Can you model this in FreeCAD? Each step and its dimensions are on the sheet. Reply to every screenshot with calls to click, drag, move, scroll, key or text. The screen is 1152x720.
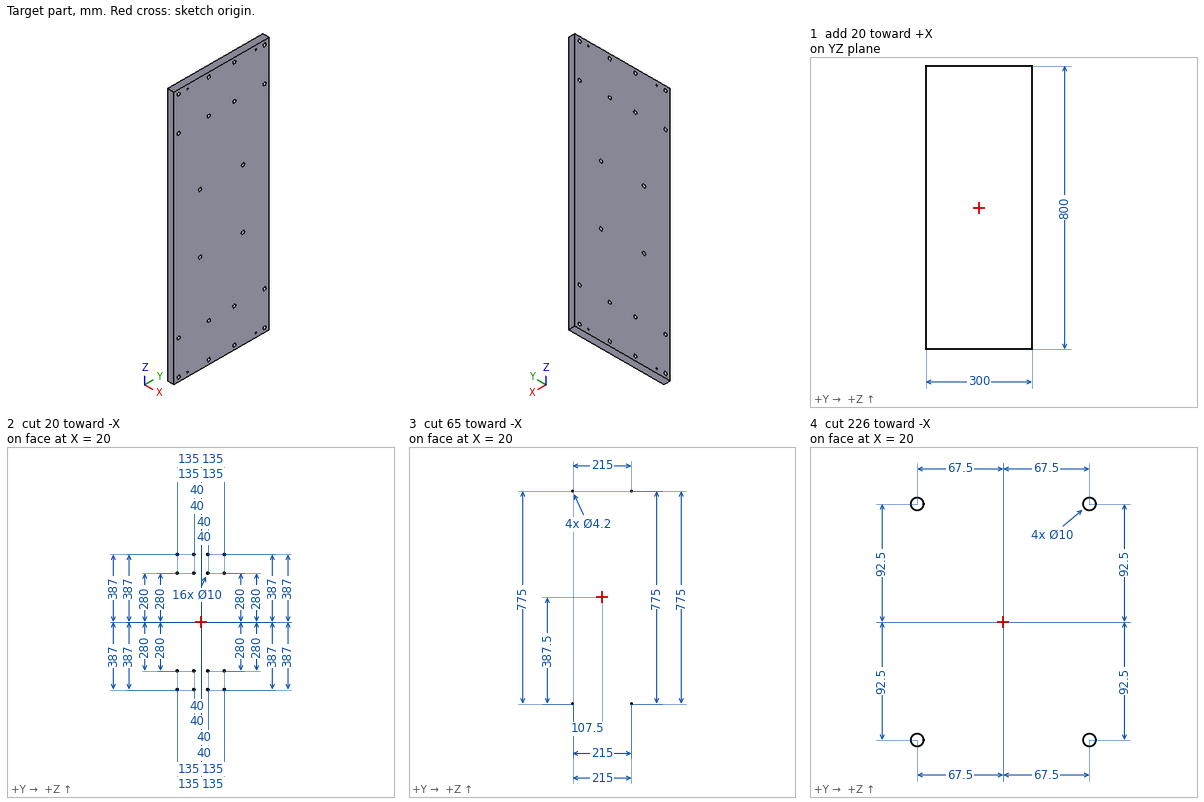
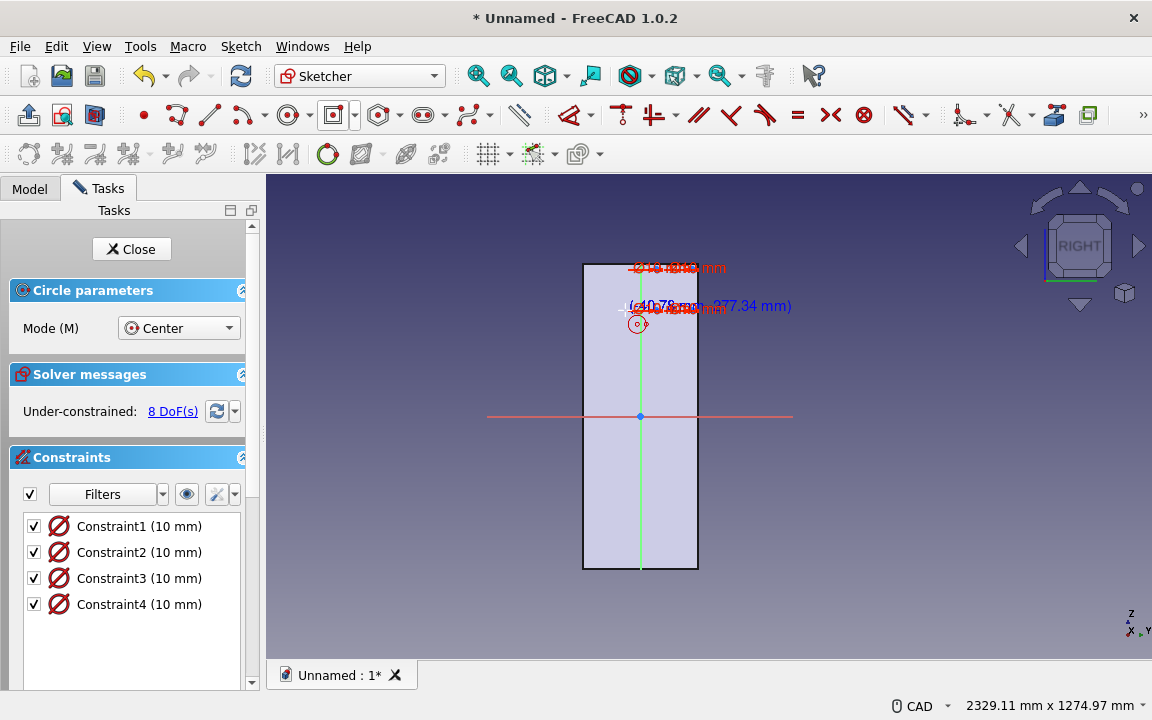
click(625, 310)
move(624, 309)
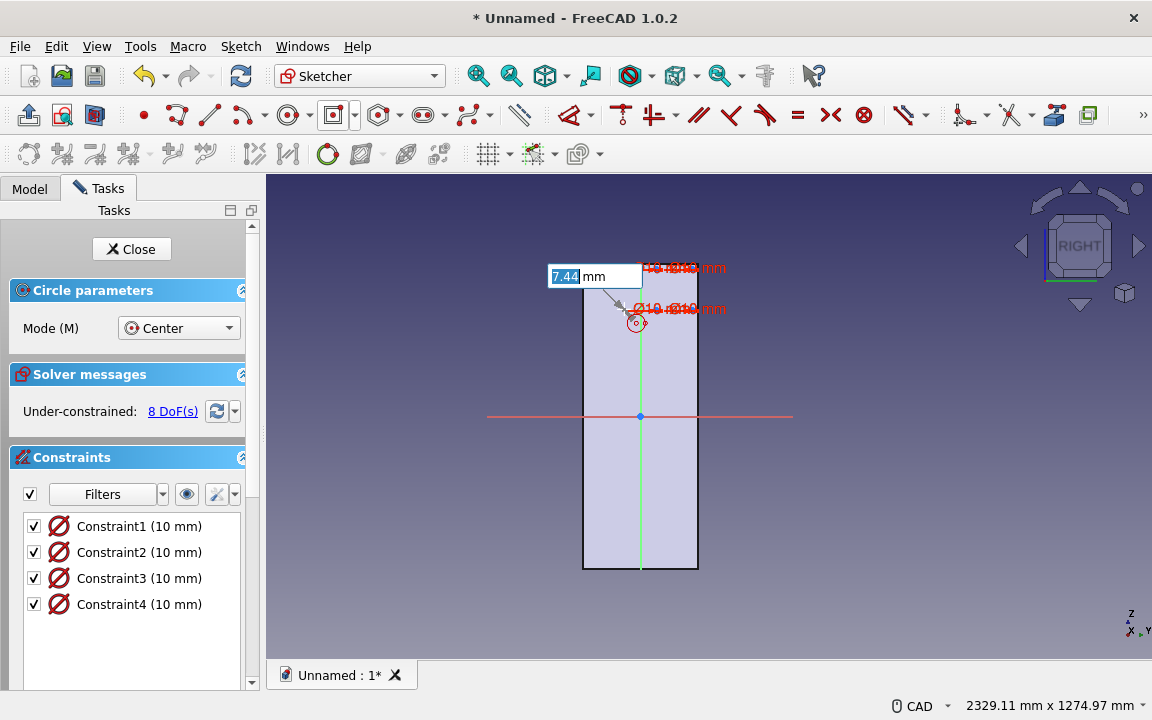
text(10)
key(Return)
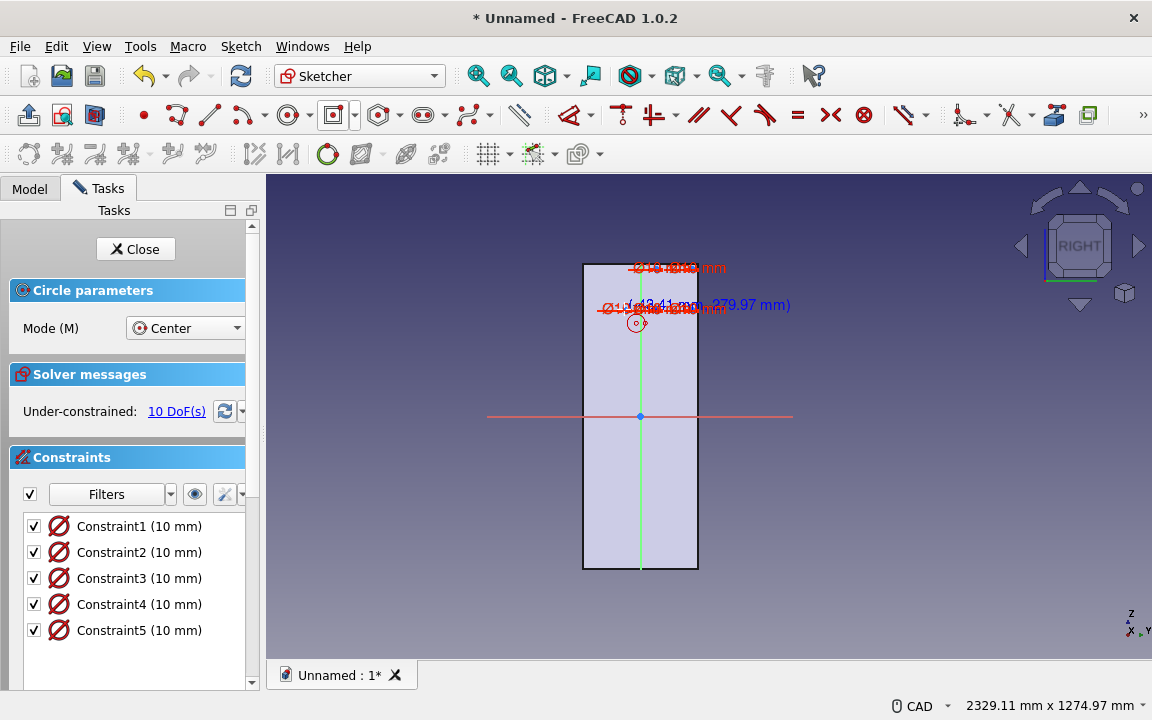
scroll(589, 310, up, 13)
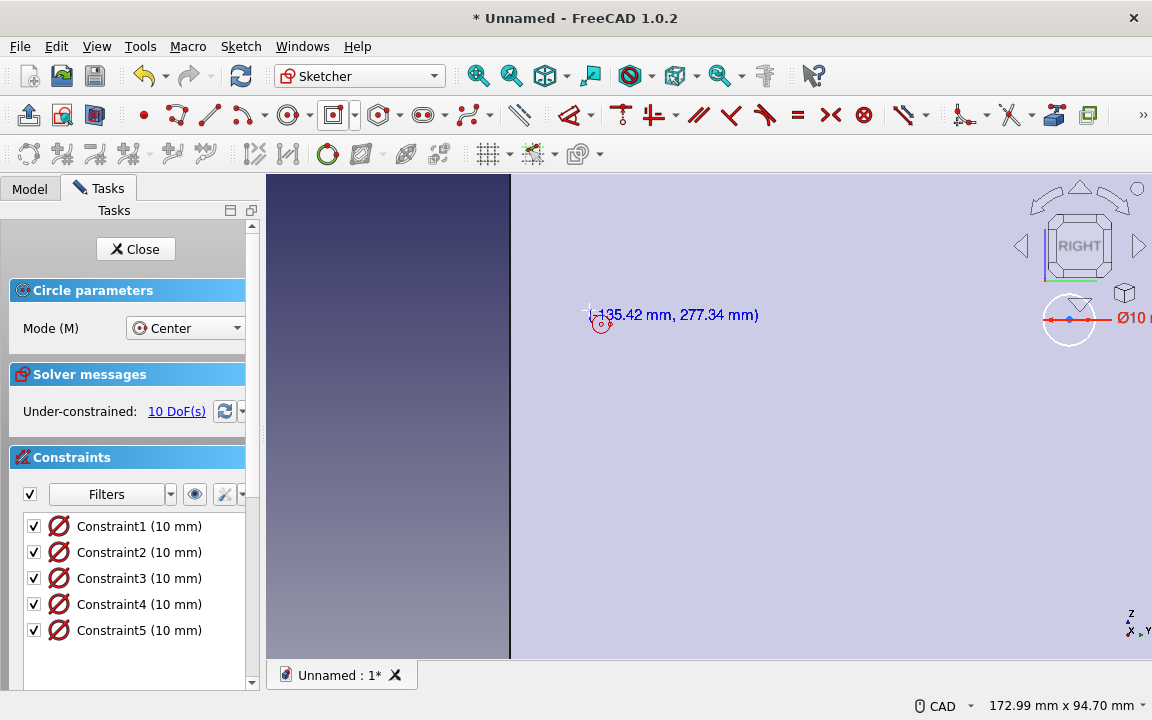
scroll(589, 310, down, 13)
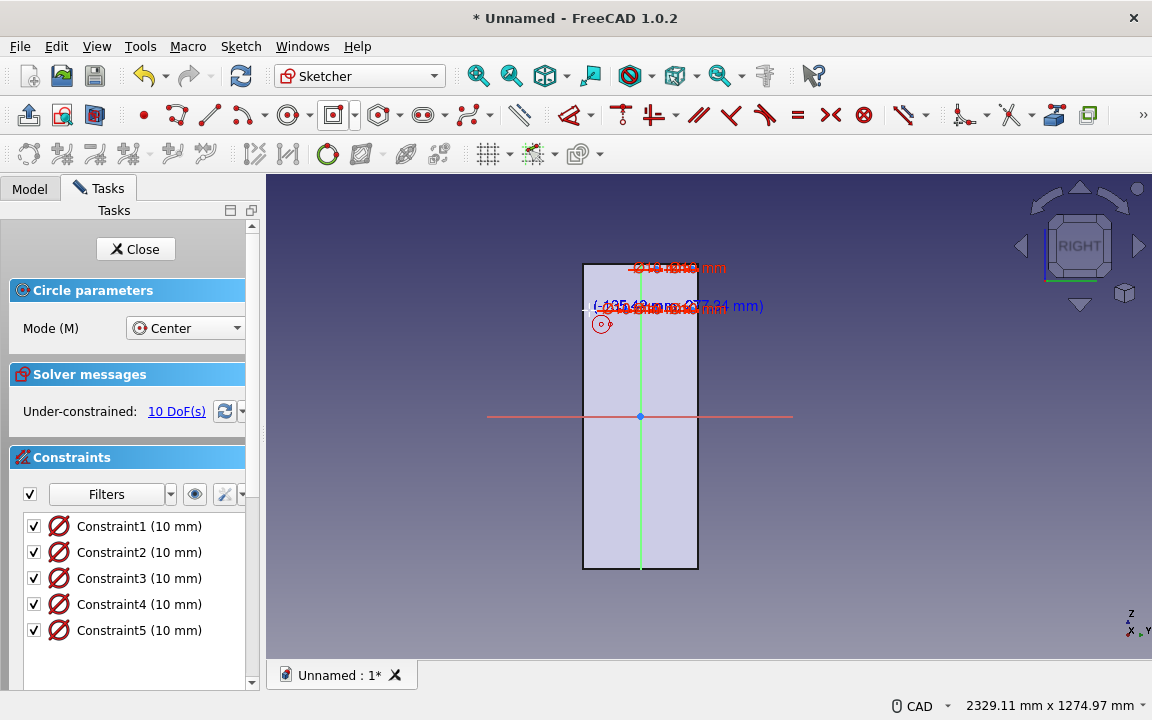
click(589, 310)
move(591, 309)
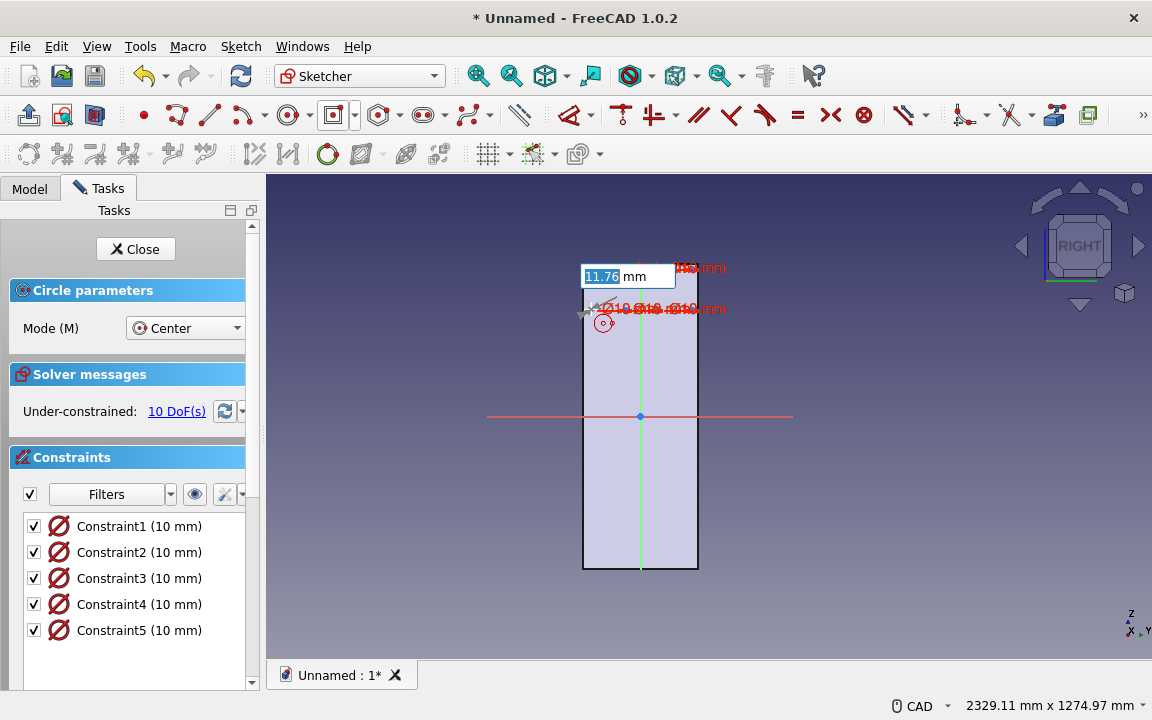
text(10)
key(Return)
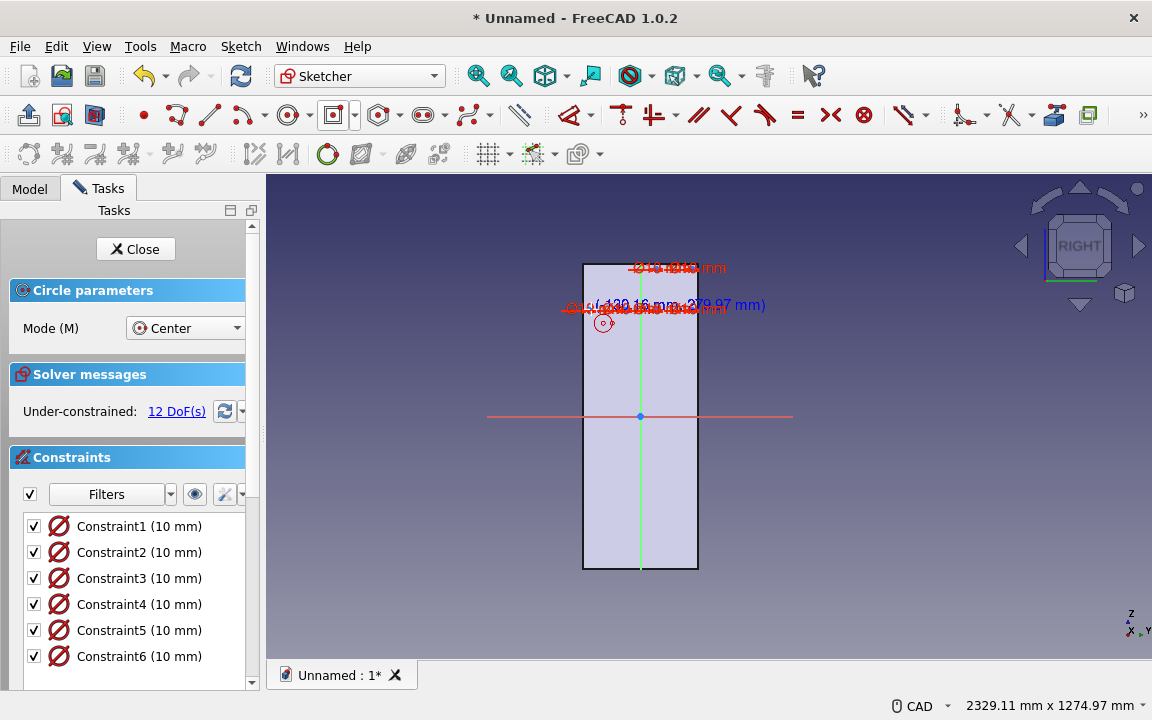
scroll(589, 269, up, 13)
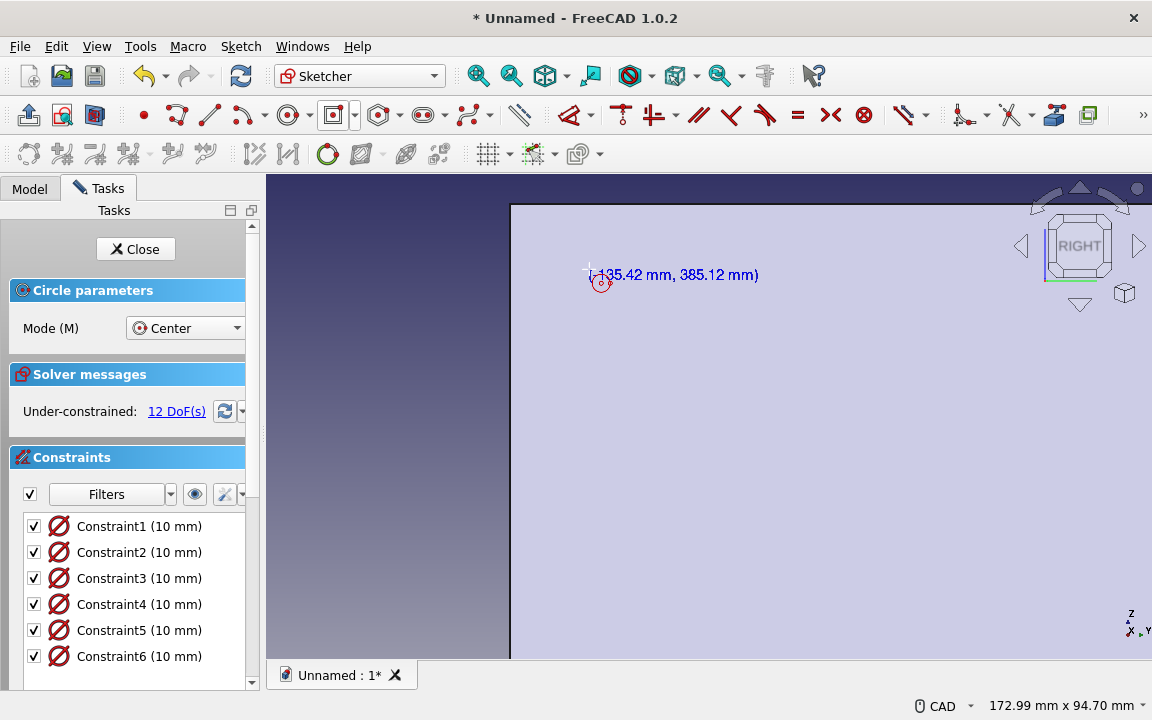
scroll(589, 269, down, 13)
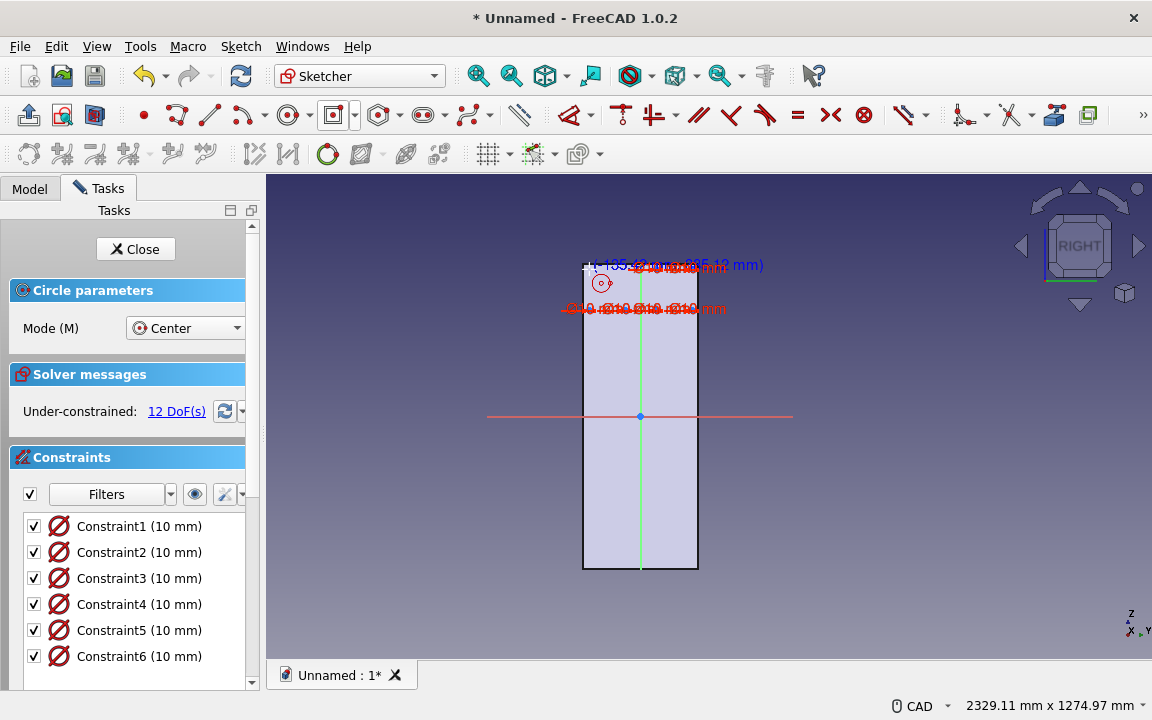
click(589, 269)
move(591, 268)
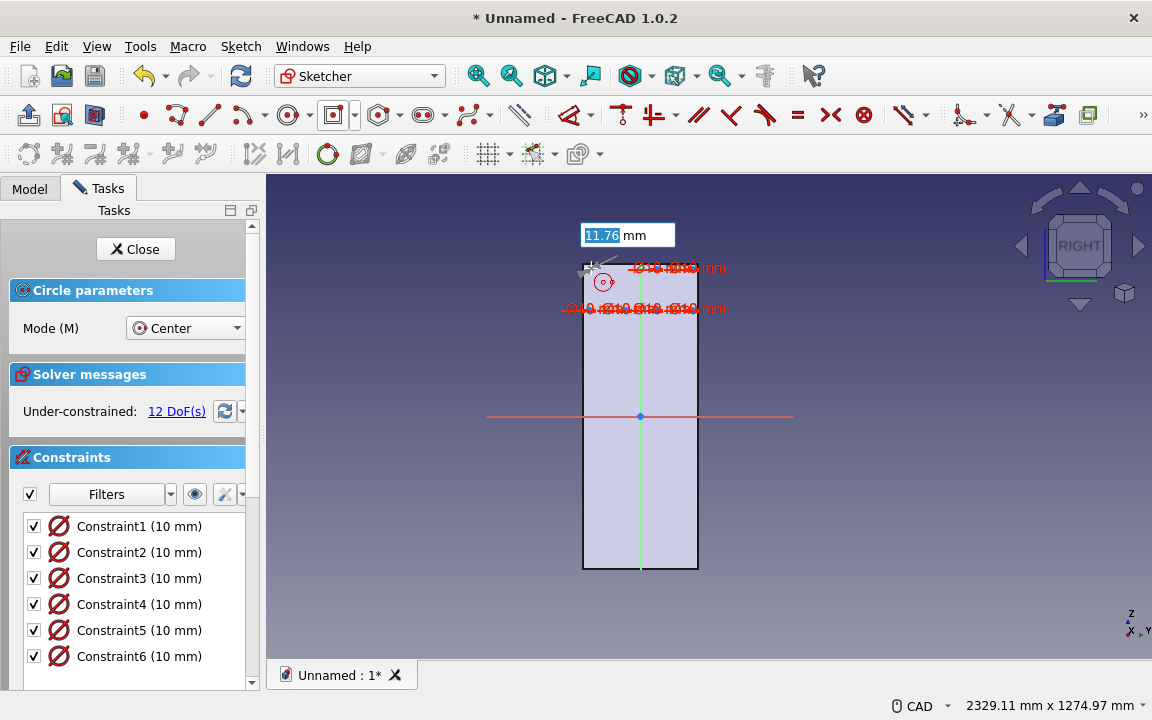
text(10)
key(Return)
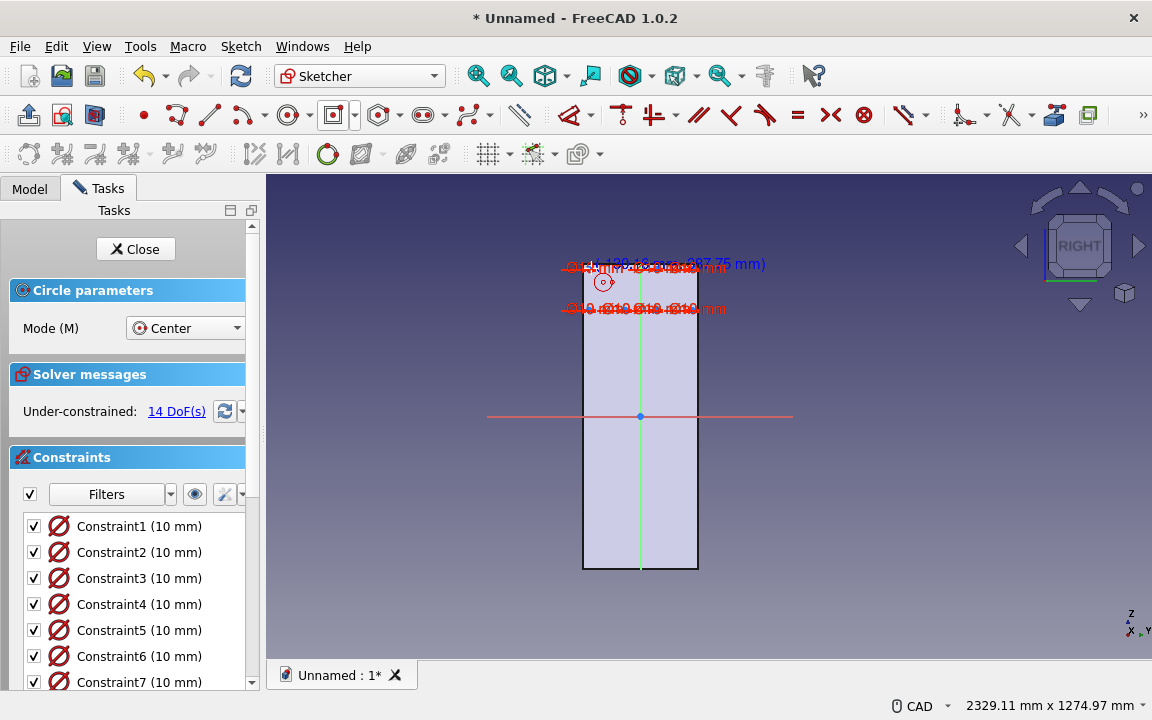
scroll(625, 269, up, 13)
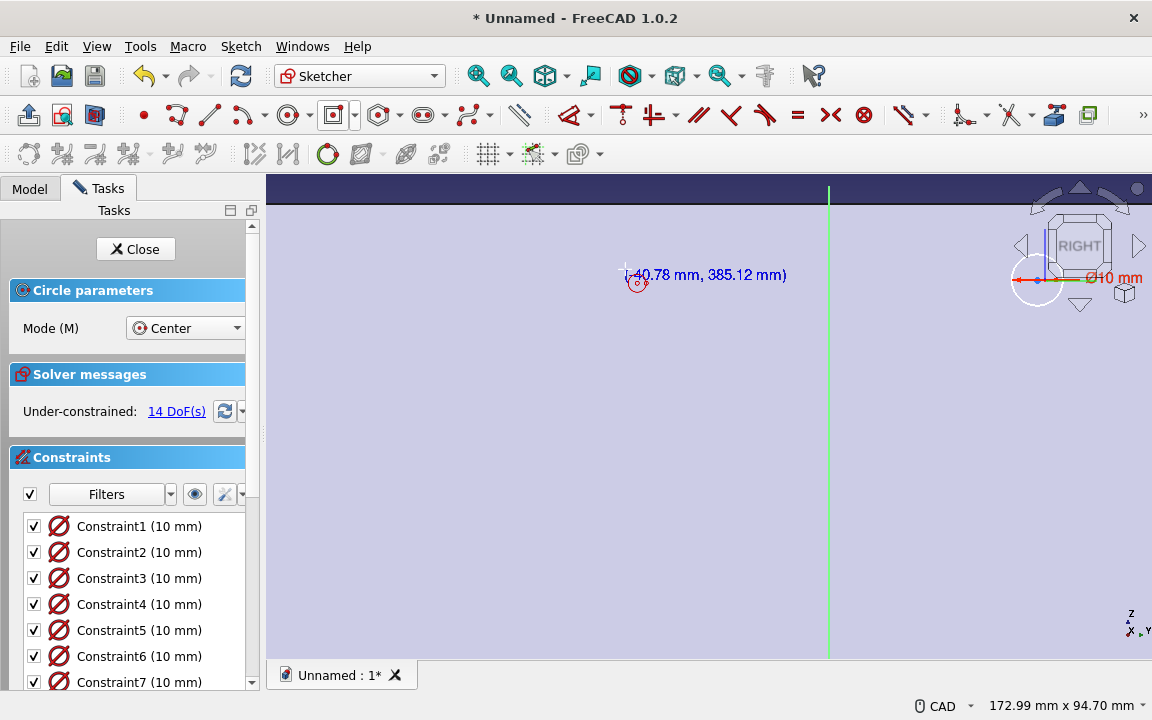
scroll(625, 269, down, 13)